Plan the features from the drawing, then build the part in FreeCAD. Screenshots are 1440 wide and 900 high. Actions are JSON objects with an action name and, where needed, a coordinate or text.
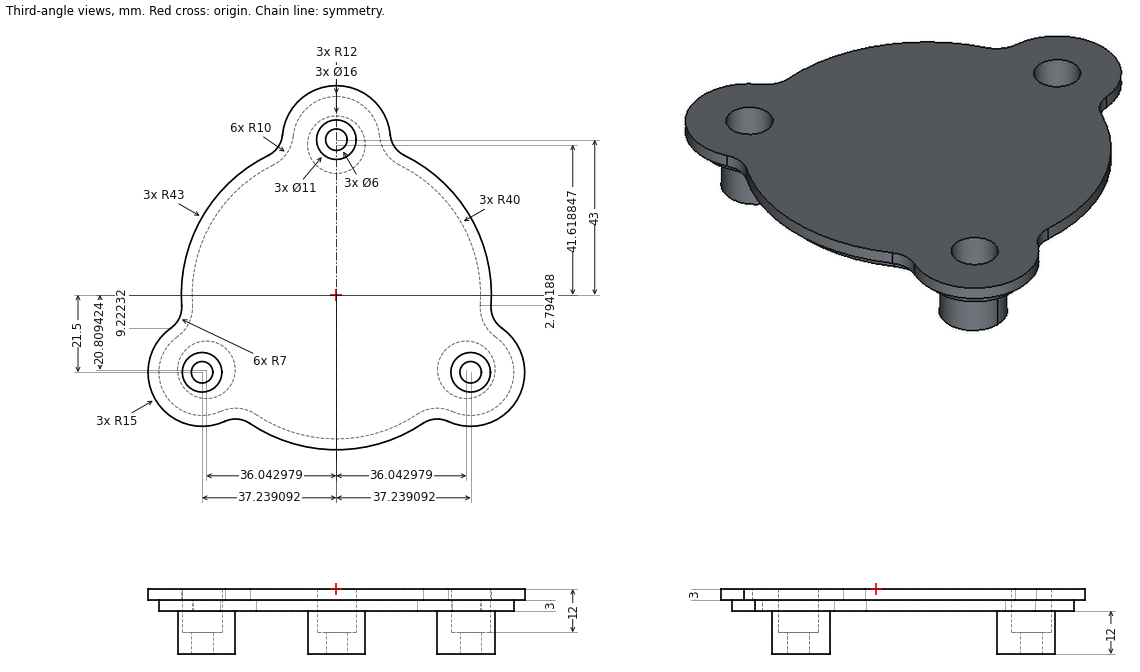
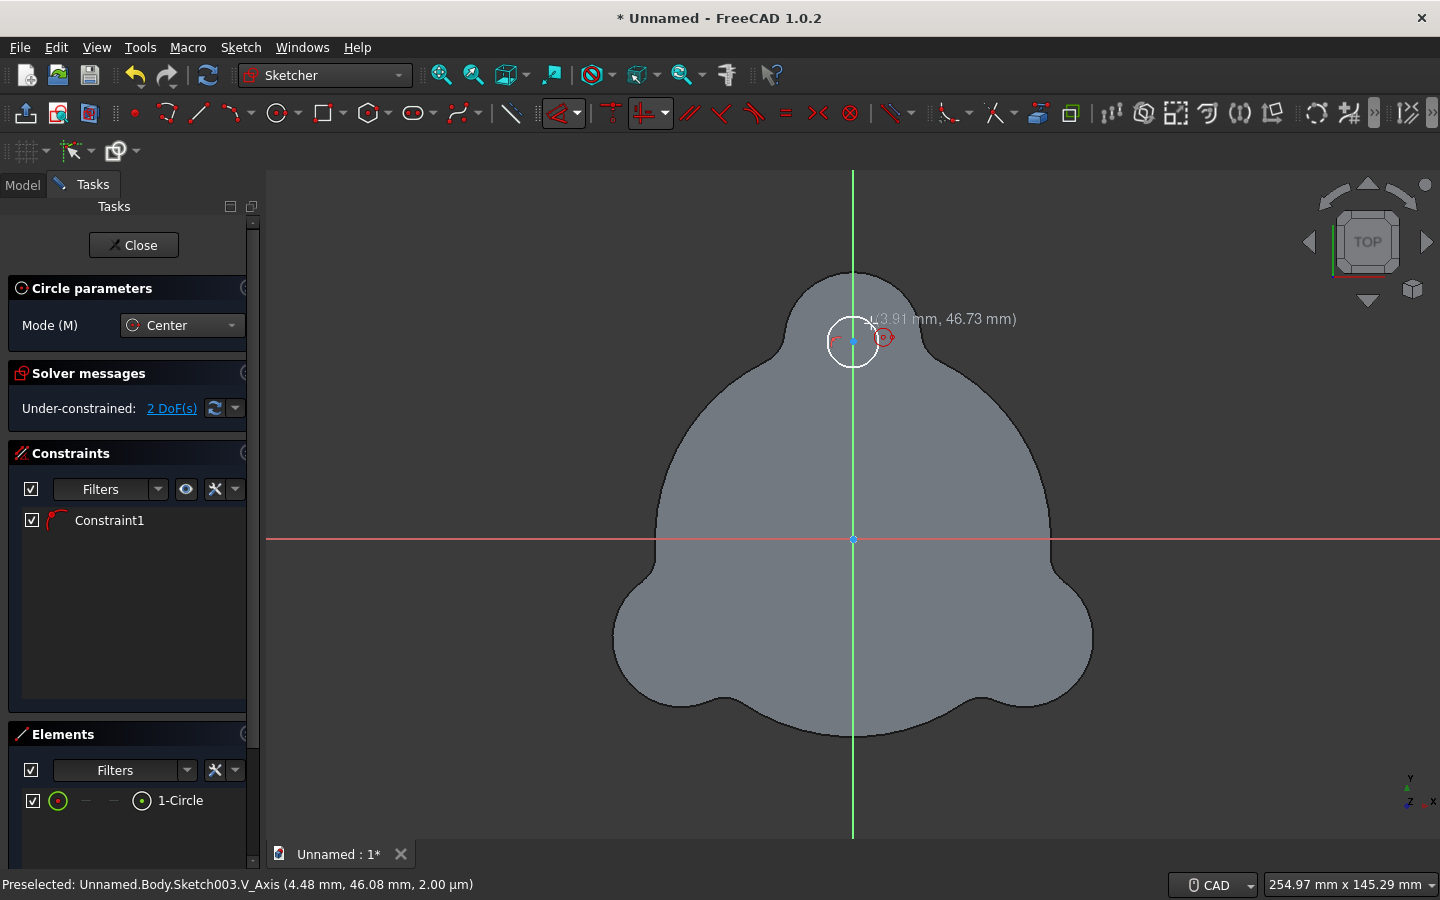
{"action": "left_click", "coordinate": [1024, 638]}
{"action": "left_click", "coordinate": [1042, 620]}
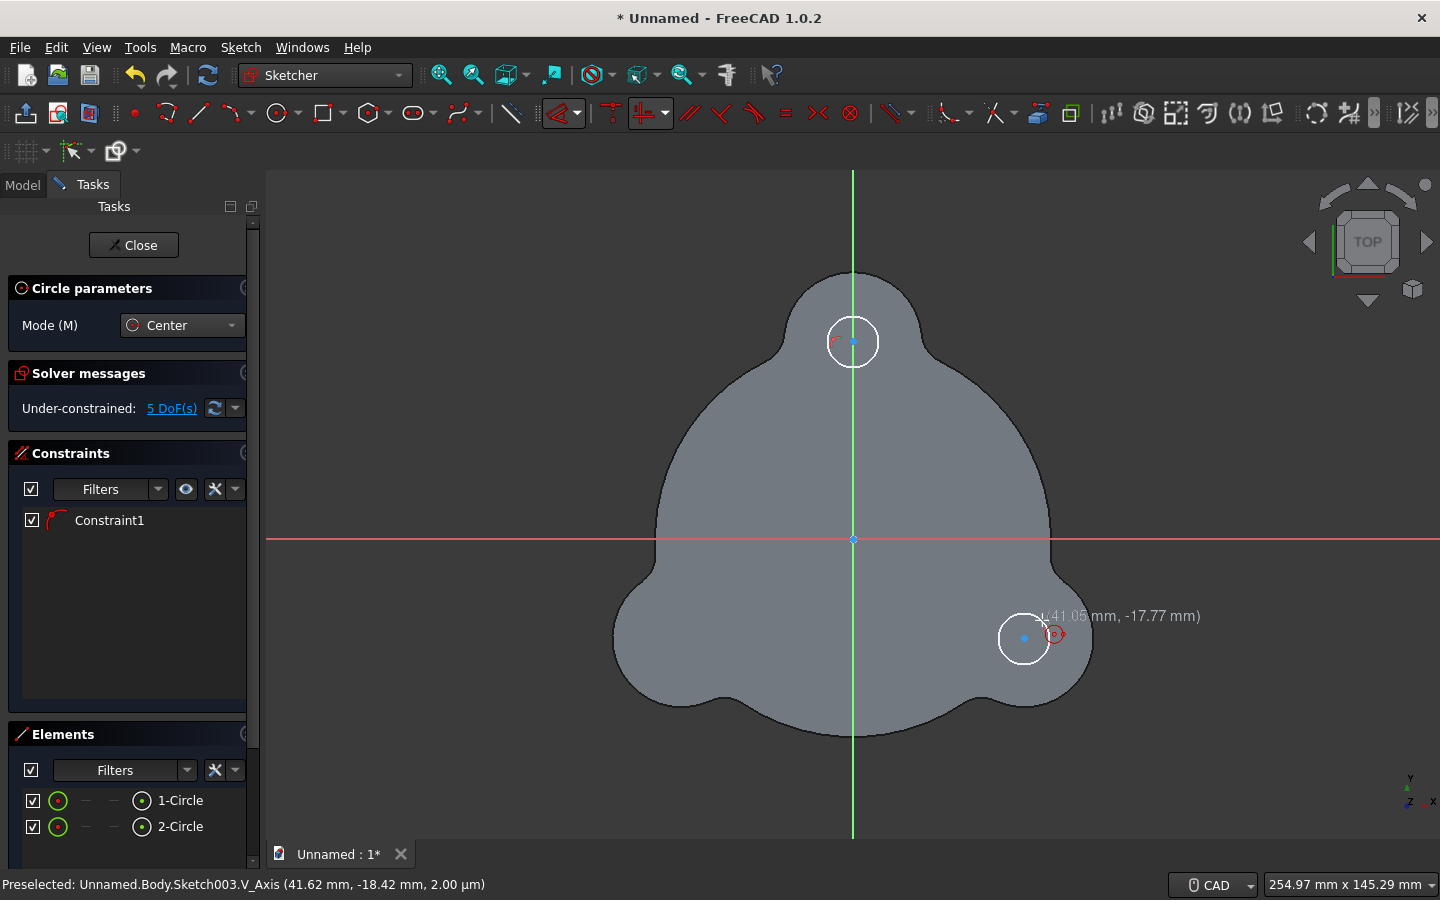
{"action": "left_click", "coordinate": [682, 638]}
{"action": "left_click", "coordinate": [699, 620]}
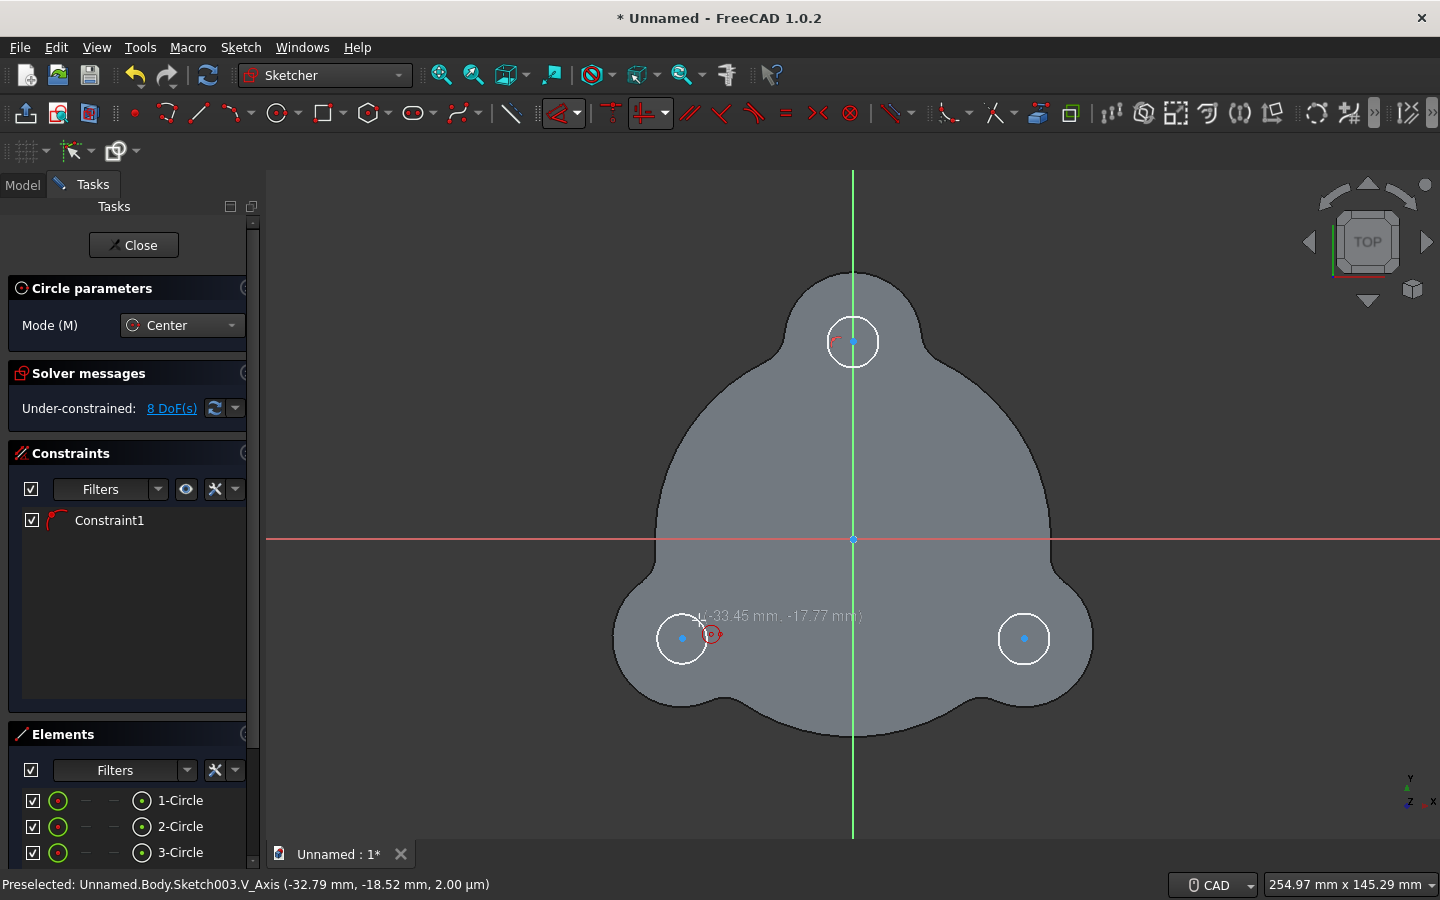
{"action": "scroll", "coordinate": [853, 341], "scroll_direction": "up", "scroll_amount": 3}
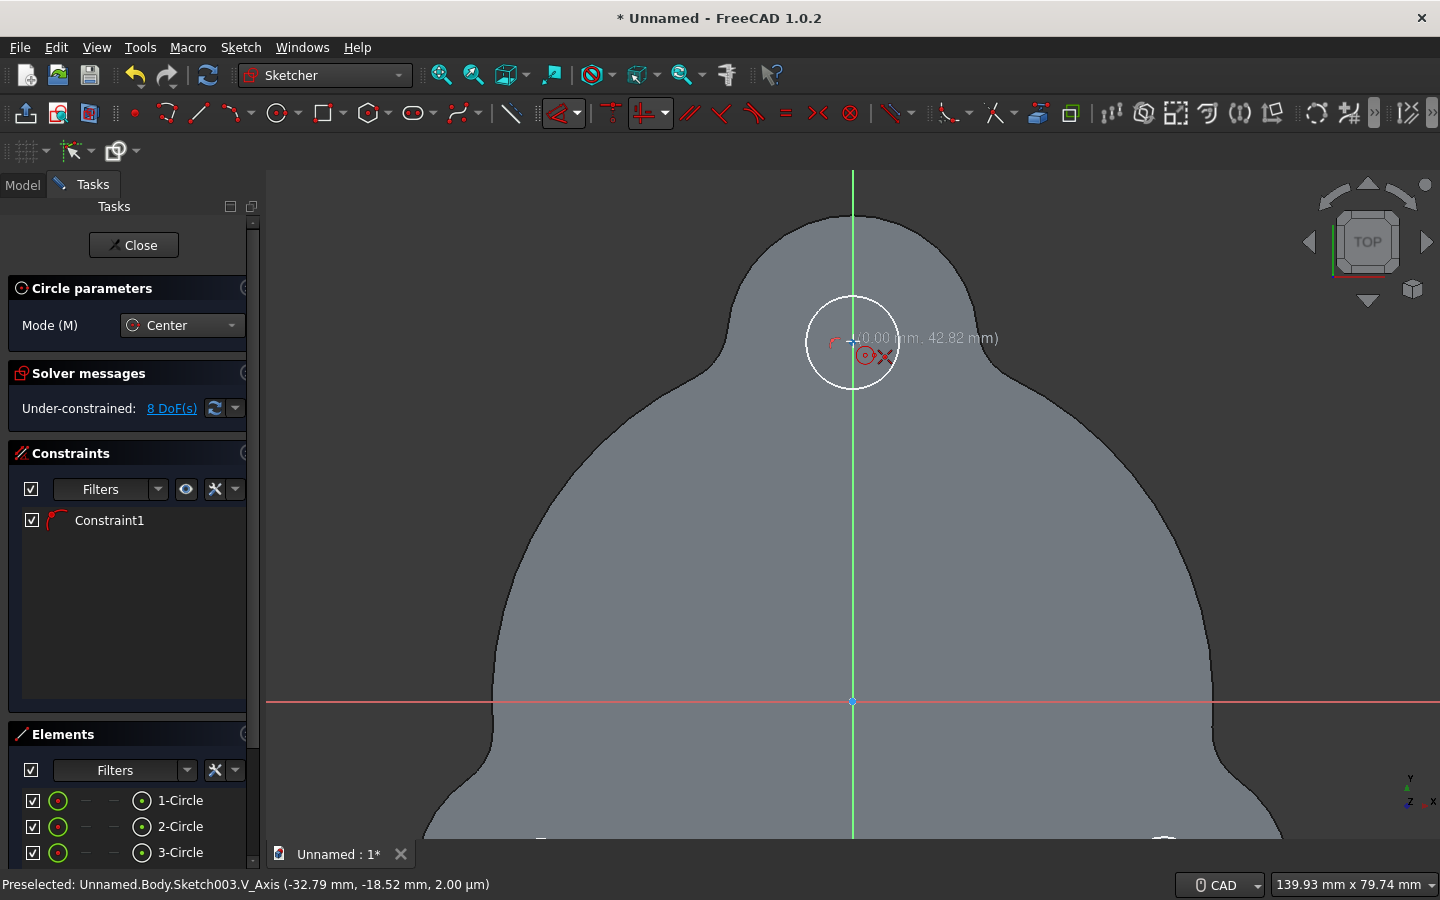
{"action": "left_click", "coordinate": [853, 343]}
{"action": "left_click", "coordinate": [870, 323]}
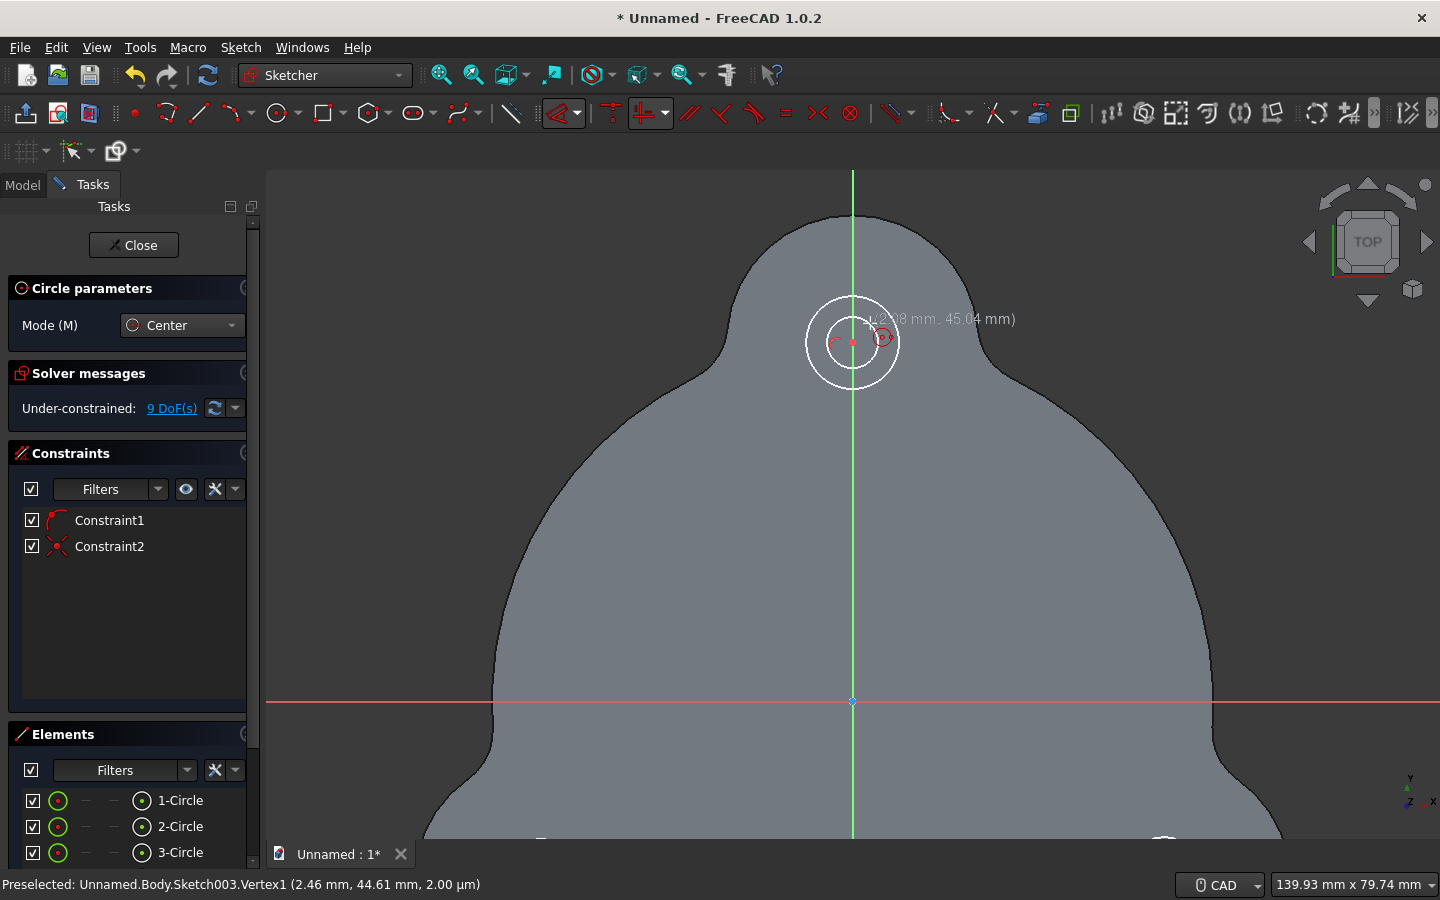
{"action": "scroll", "coordinate": [646, 287], "scroll_direction": "down", "scroll_amount": 2}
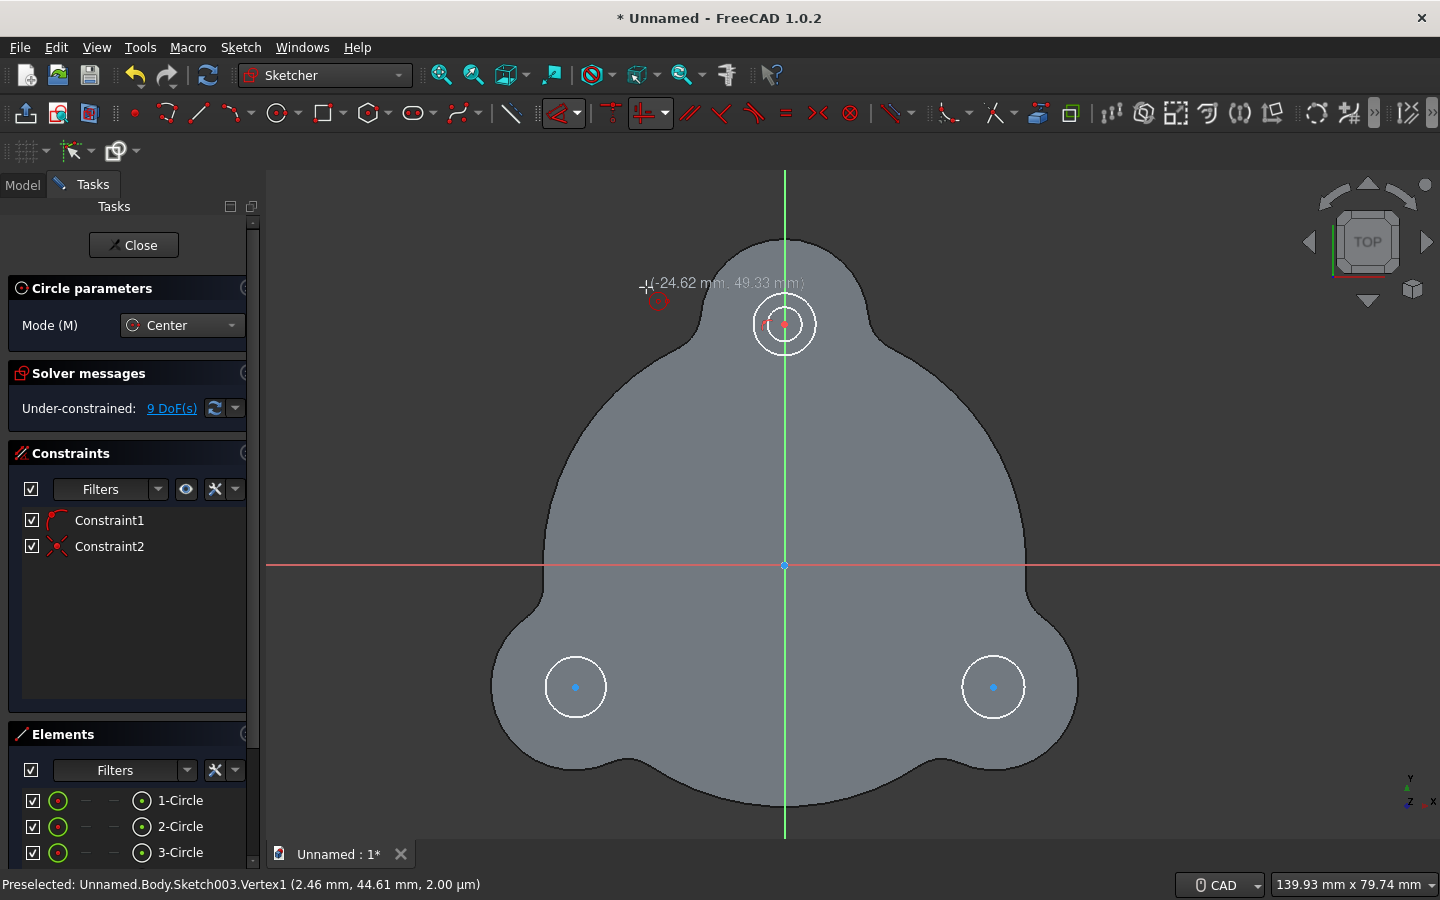
{"action": "scroll", "coordinate": [994, 686], "scroll_direction": "up", "scroll_amount": 2}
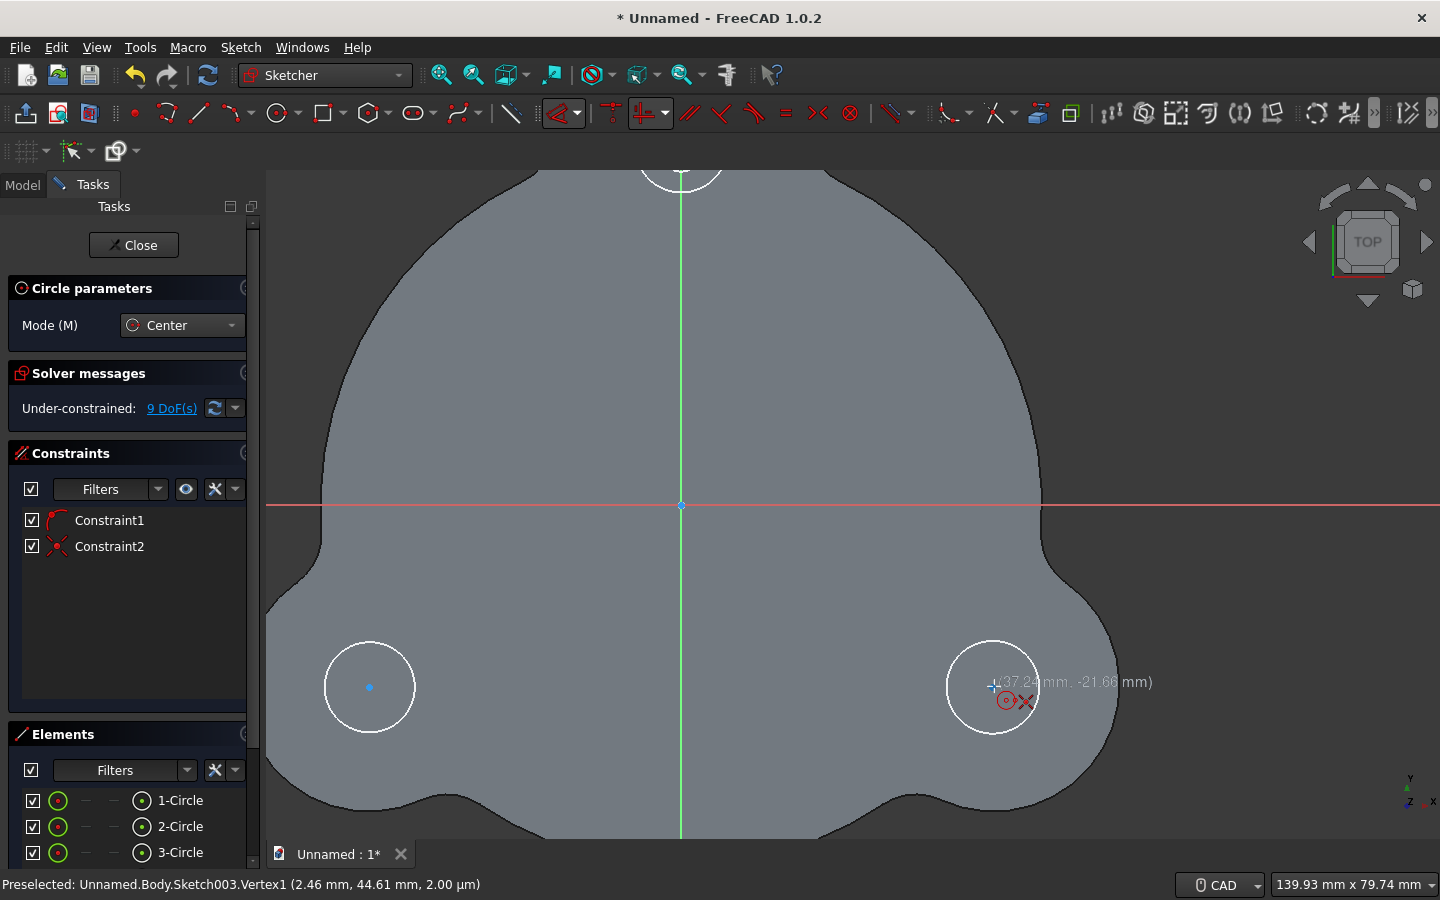
{"action": "left_click", "coordinate": [993, 687]}
{"action": "left_click", "coordinate": [1012, 668]}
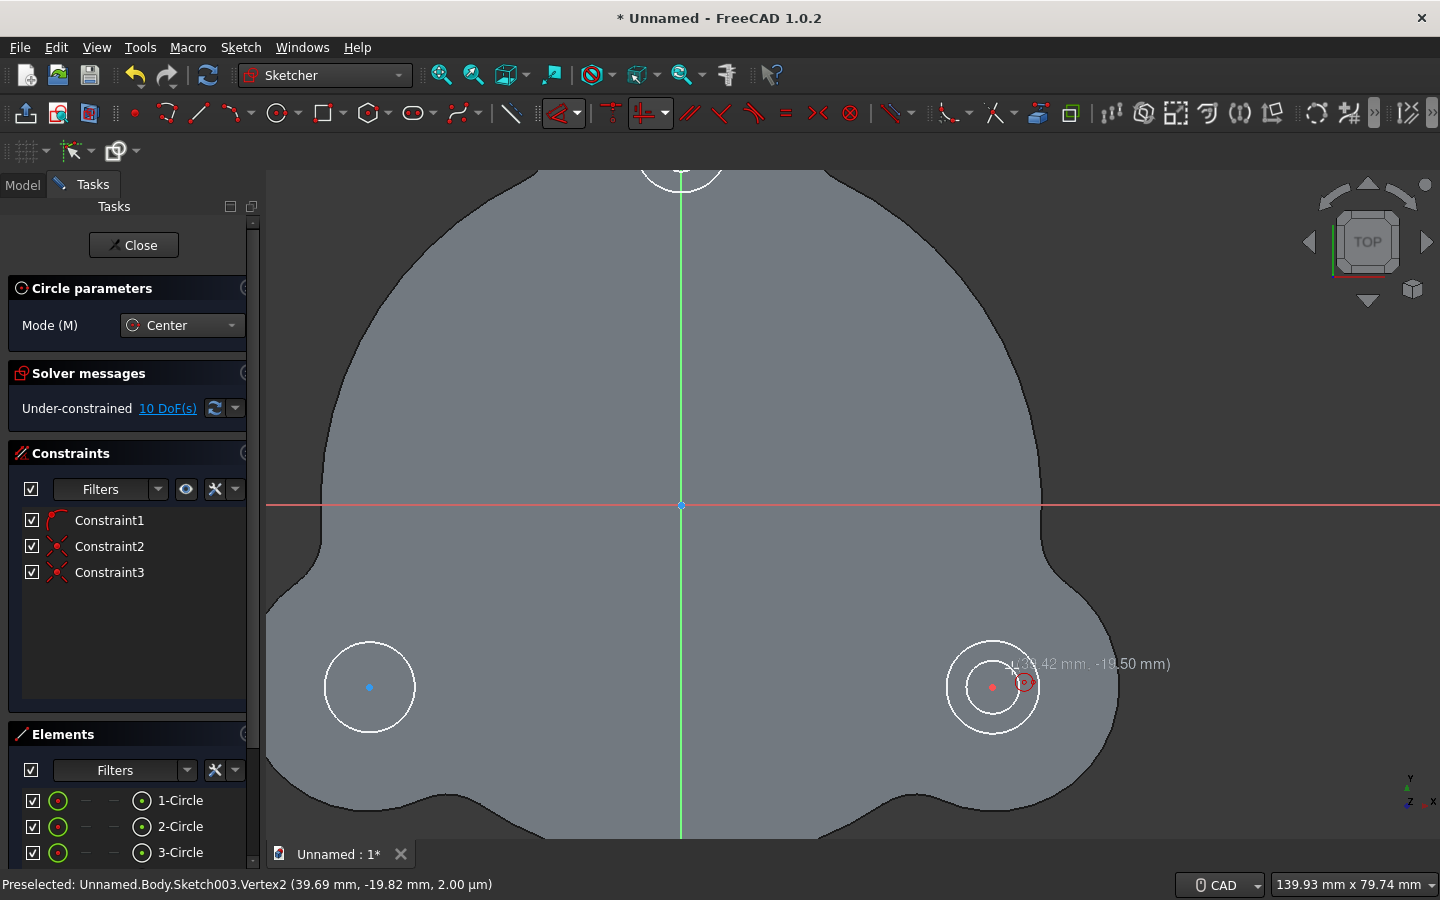
{"action": "left_click", "coordinate": [370, 687]}
{"action": "left_click", "coordinate": [387, 668]}
{"action": "key", "text": "Escape"}